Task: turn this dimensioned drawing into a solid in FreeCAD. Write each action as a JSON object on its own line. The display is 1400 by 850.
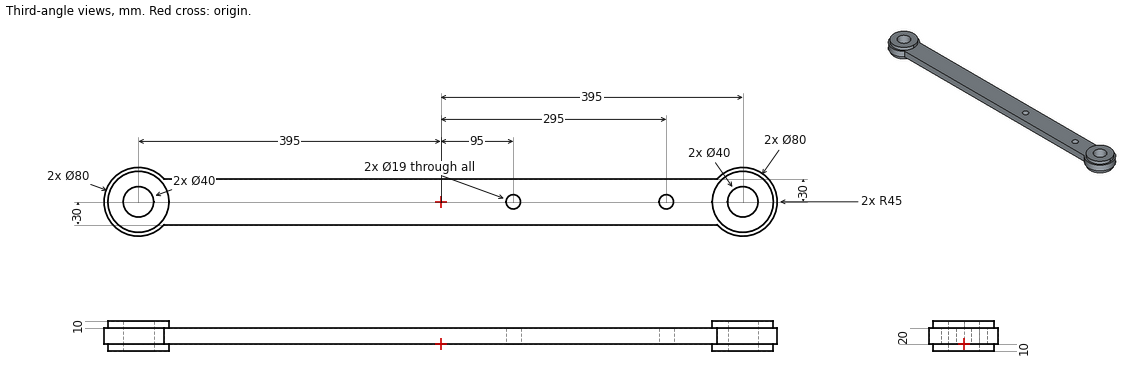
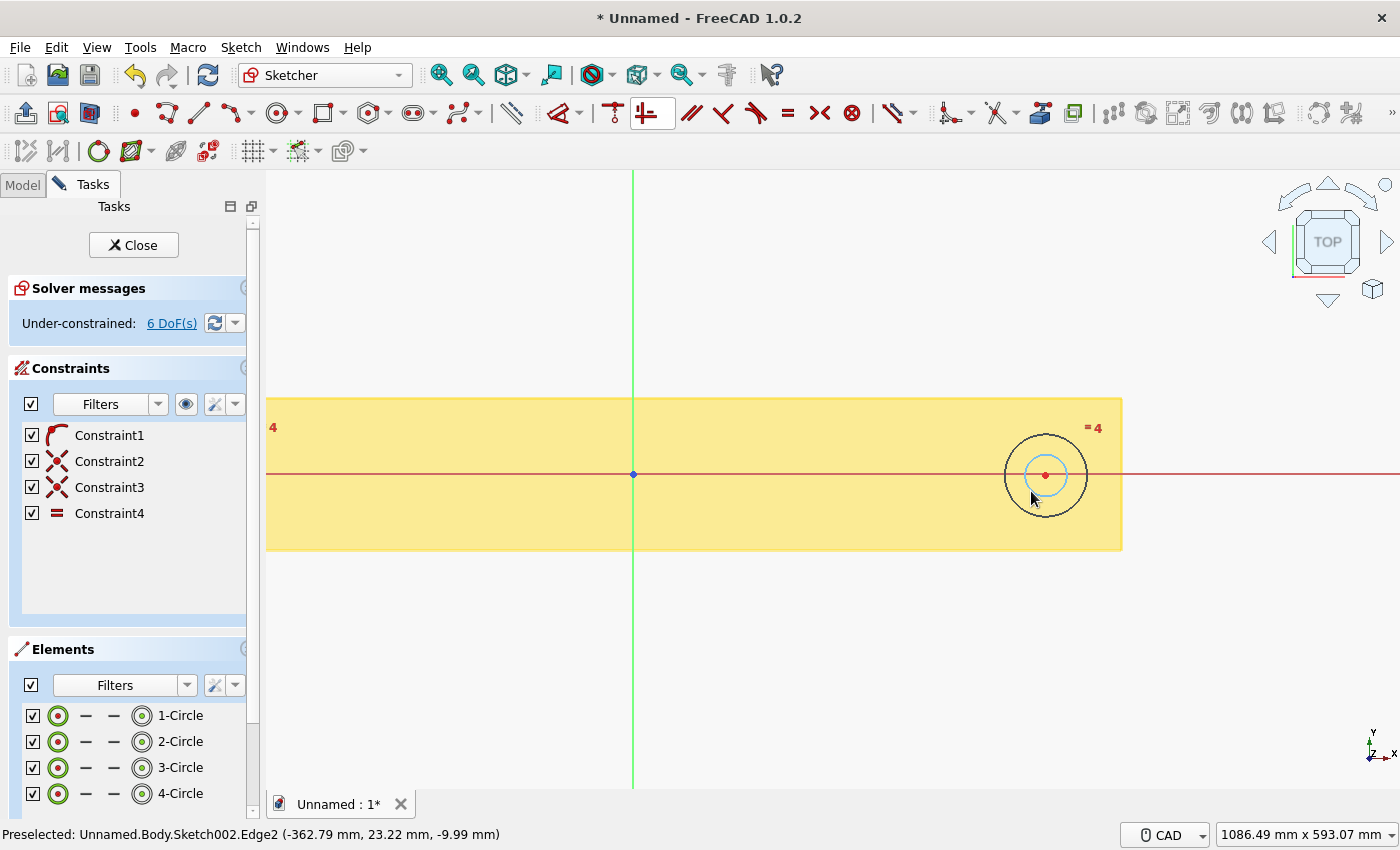
{"action": "left_click", "coordinate": [1031, 490]}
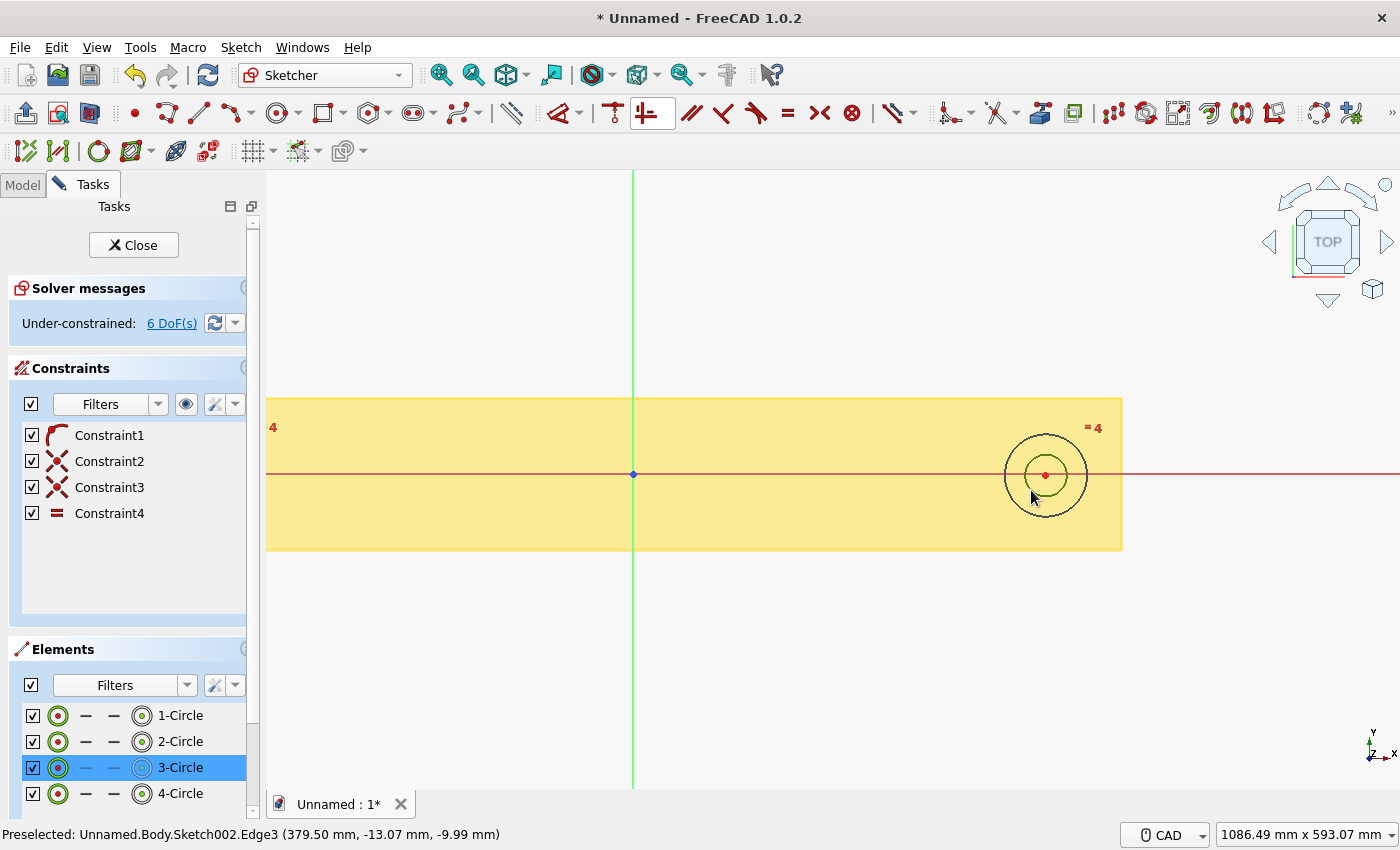
{"action": "scroll", "coordinate": [1032, 490], "scroll_direction": "down", "scroll_amount": 2}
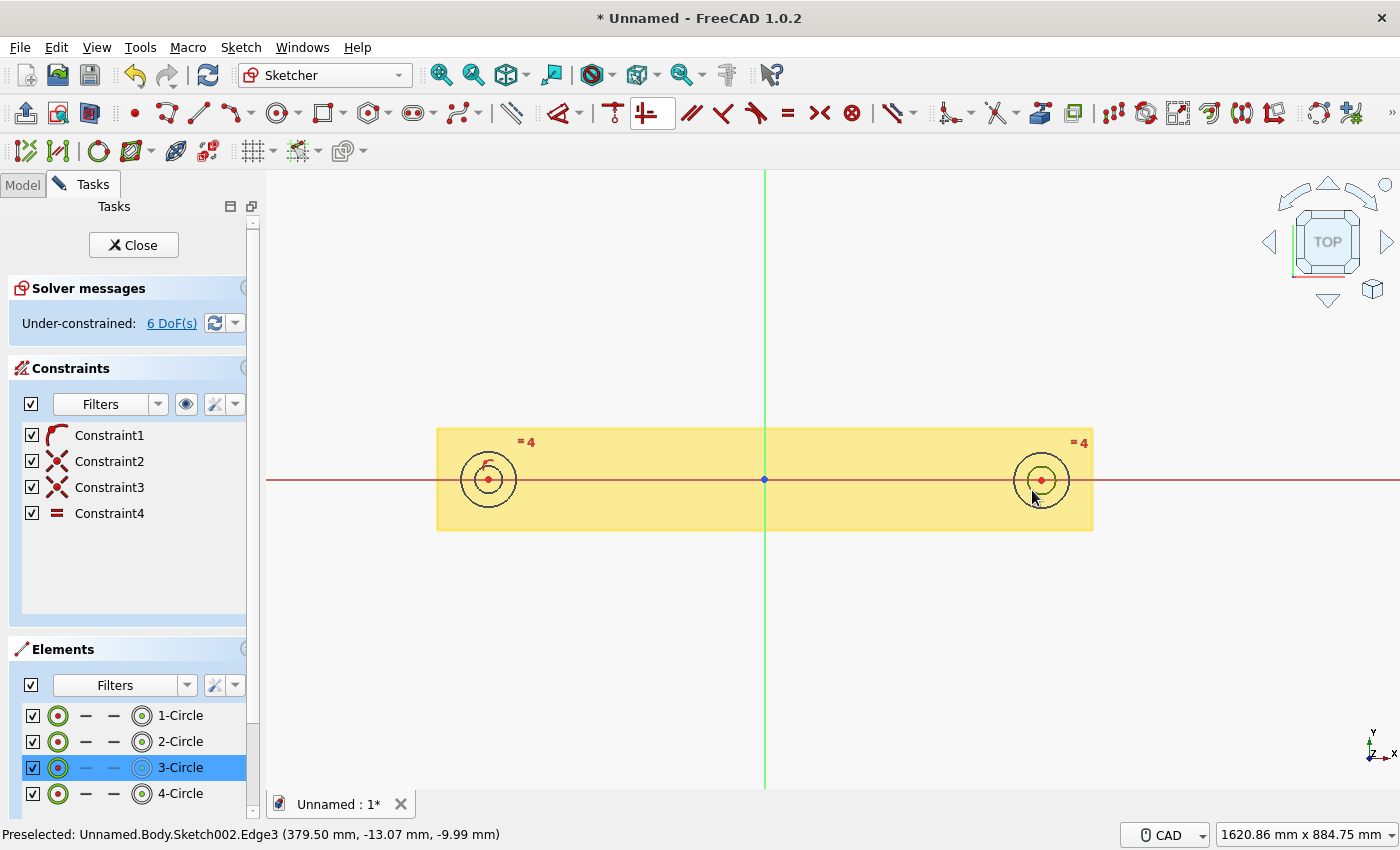
{"action": "scroll", "coordinate": [498, 470], "scroll_direction": "up", "scroll_amount": 2}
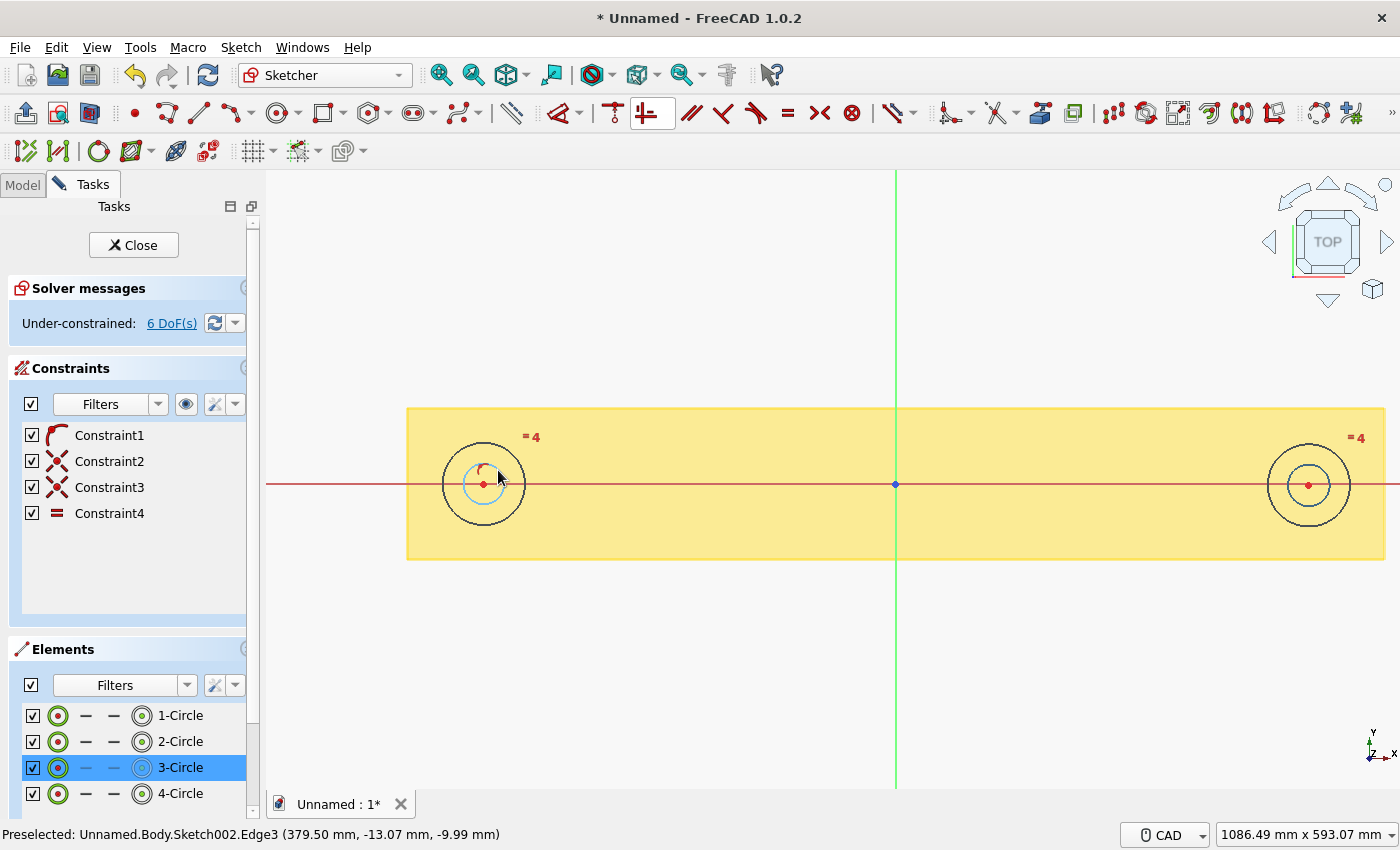
{"action": "left_click", "coordinate": [498, 470]}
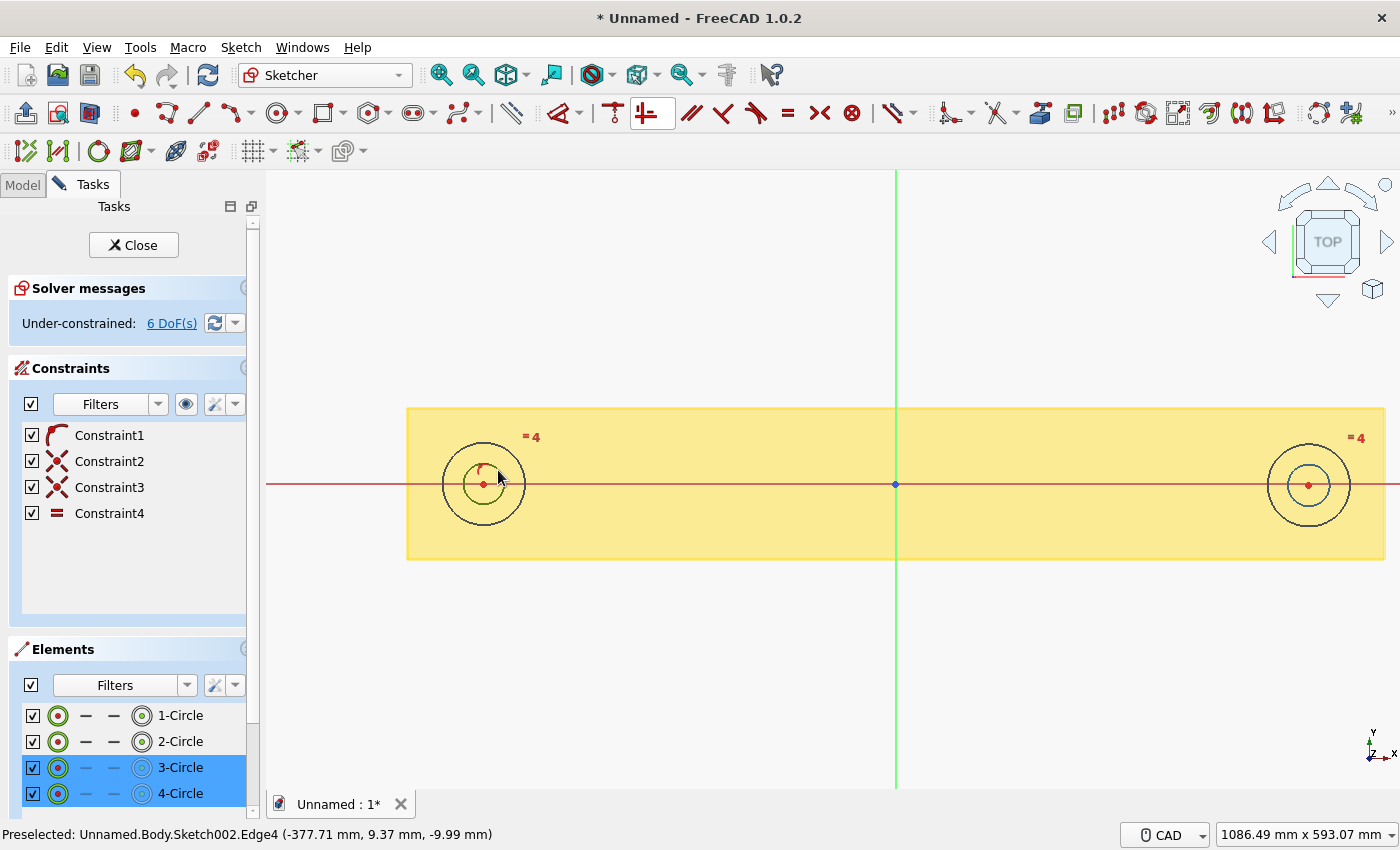
{"action": "key", "text": "e"}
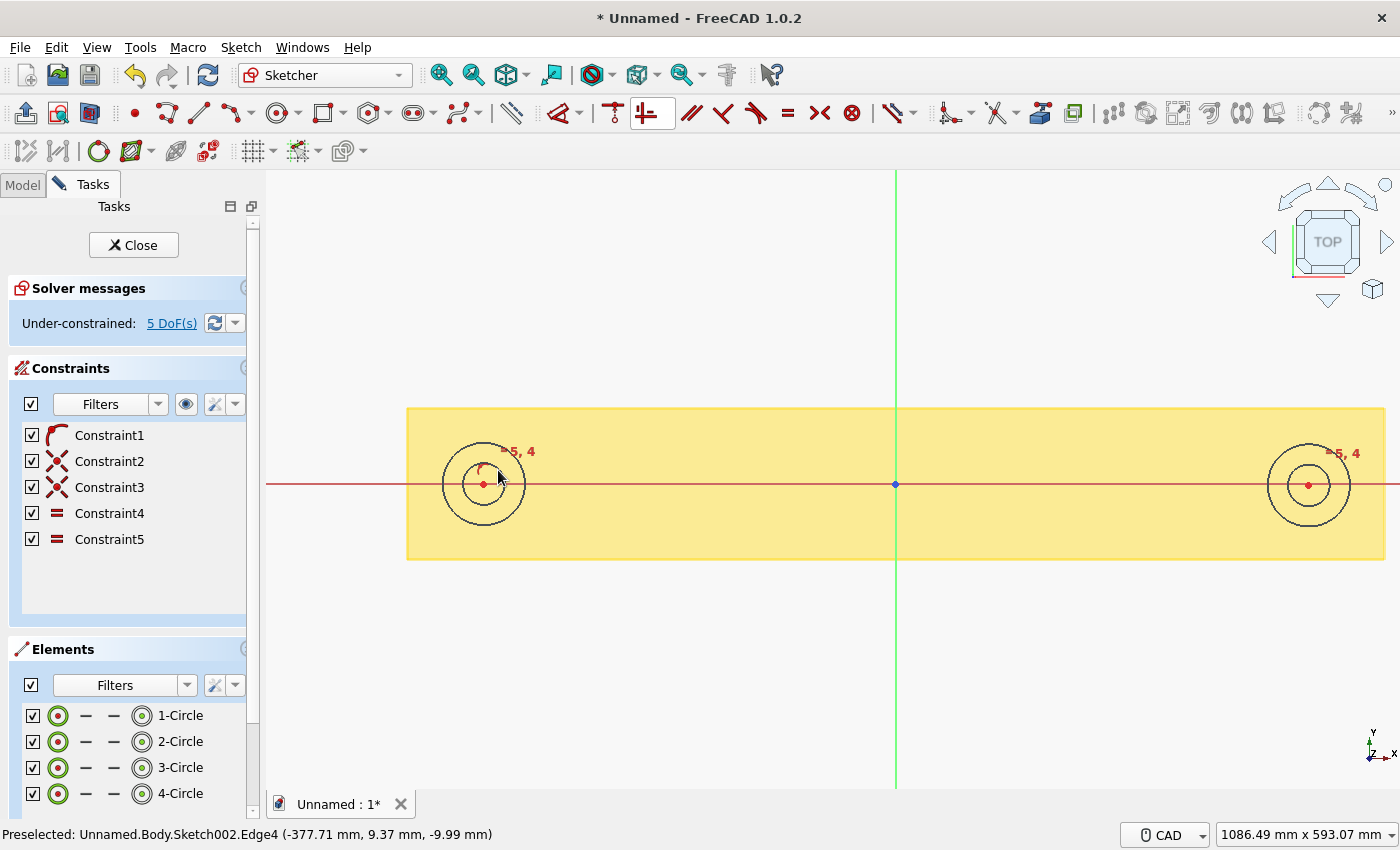
{"action": "scroll", "coordinate": [497, 470], "scroll_direction": "down", "scroll_amount": 2}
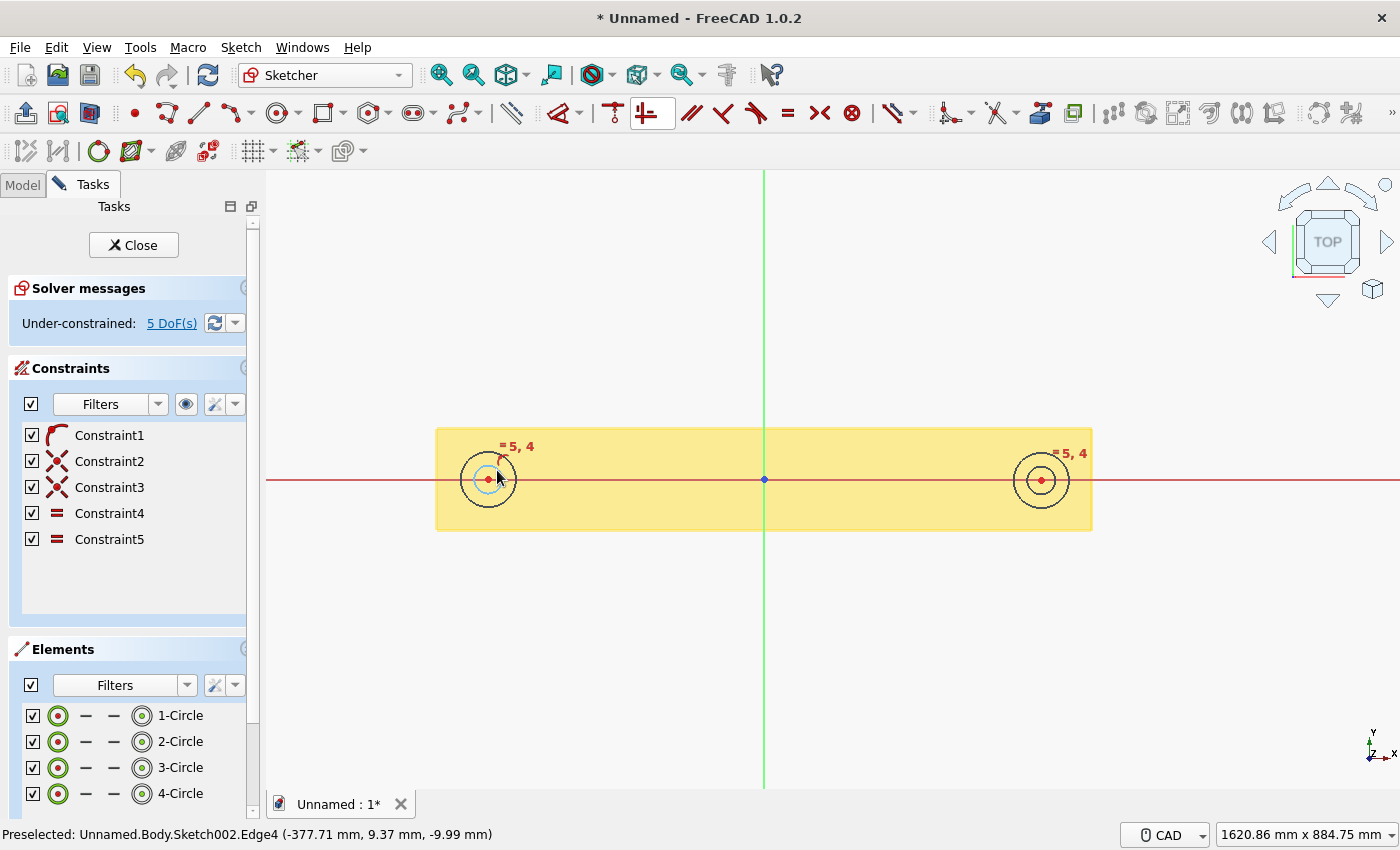
{"action": "left_click", "coordinate": [1041, 480]}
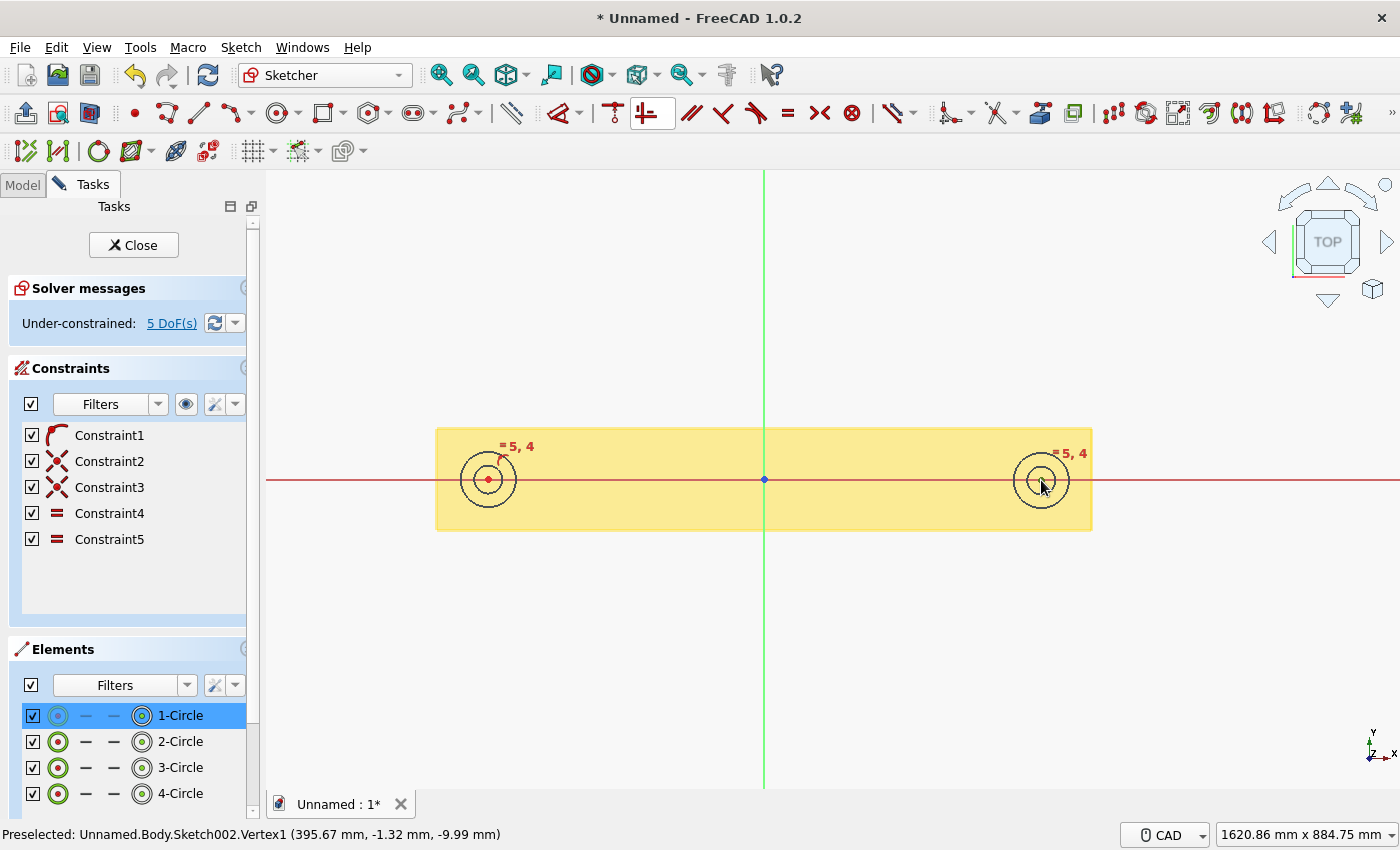
{"action": "left_click", "coordinate": [361, 480]}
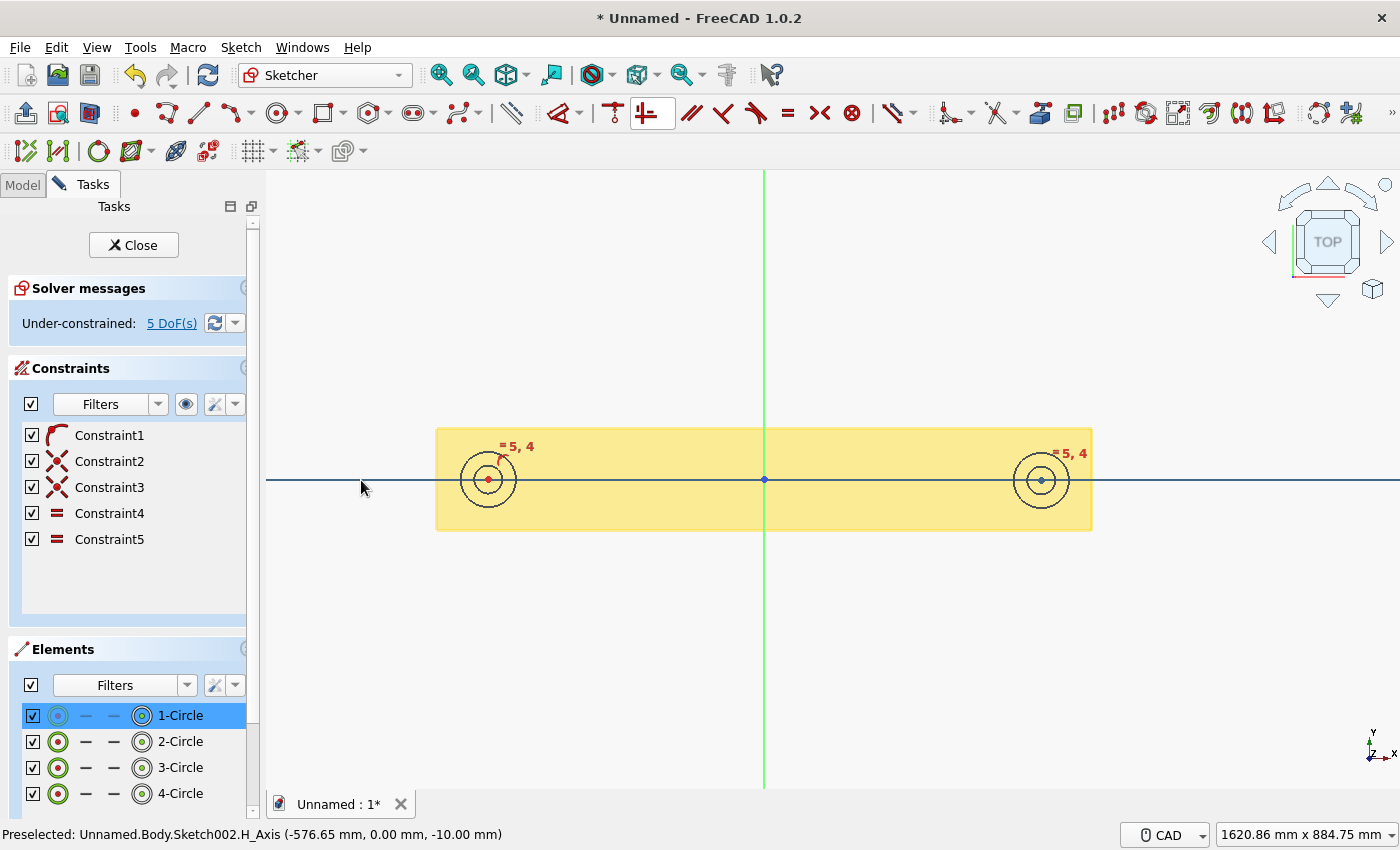
{"action": "left_click", "coordinate": [614, 114]}